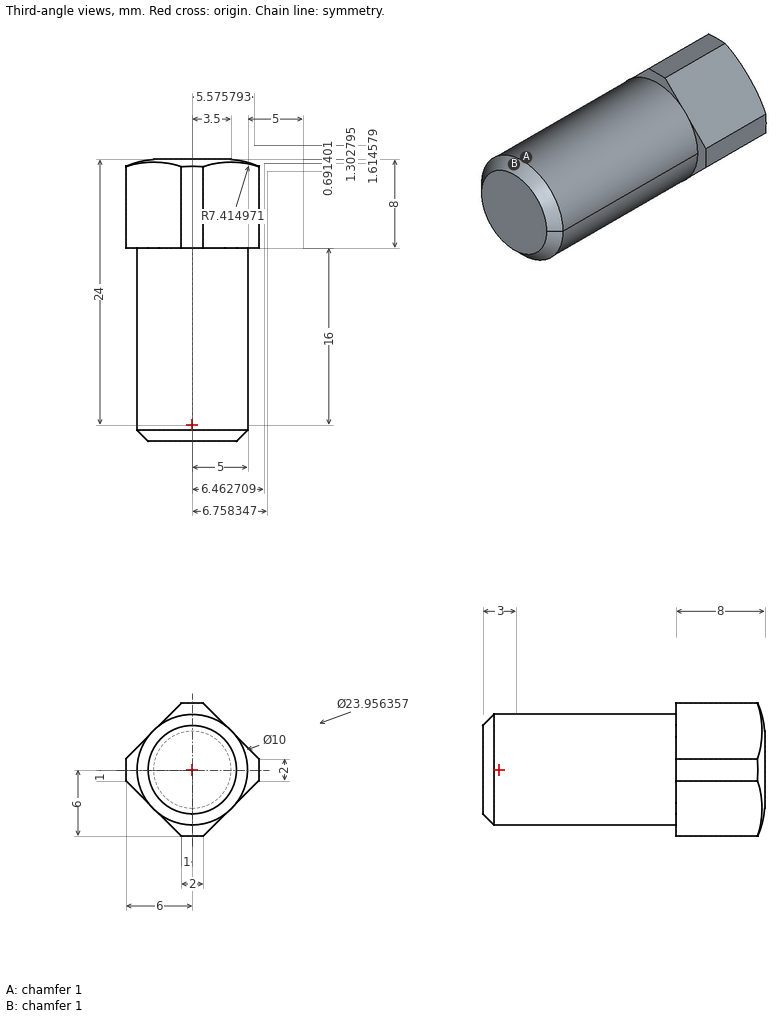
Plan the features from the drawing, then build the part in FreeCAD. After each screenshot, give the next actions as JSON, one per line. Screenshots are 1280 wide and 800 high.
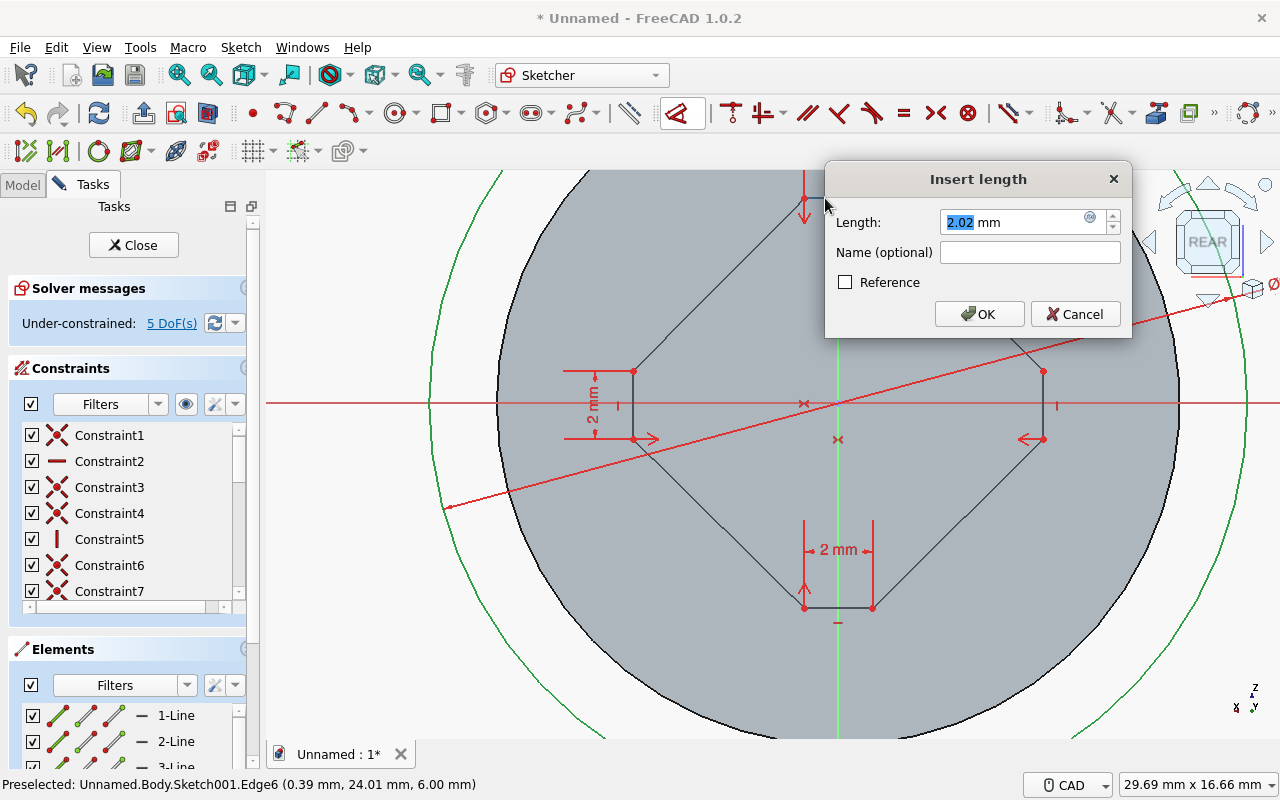
{"action": "type", "text": "2"}
{"action": "key", "text": "Return"}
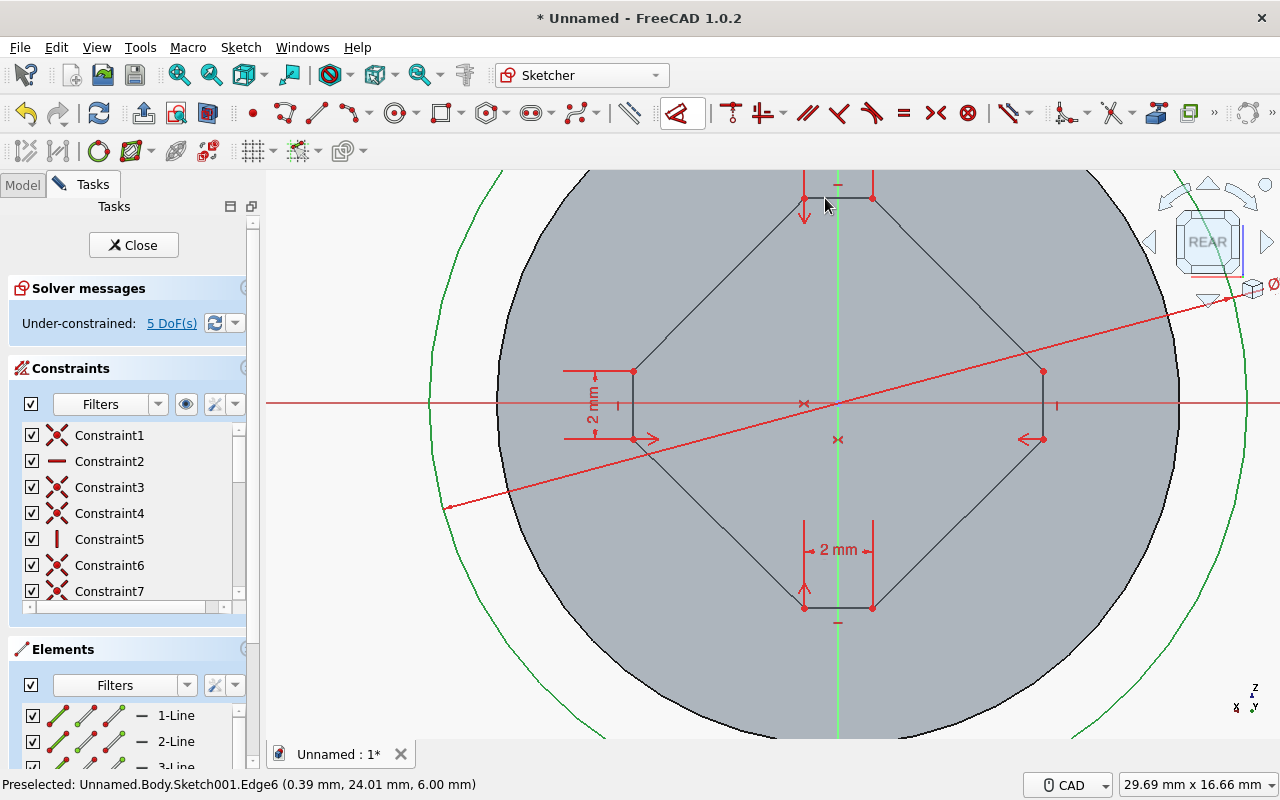
{"action": "left_click", "coordinate": [1043, 392]}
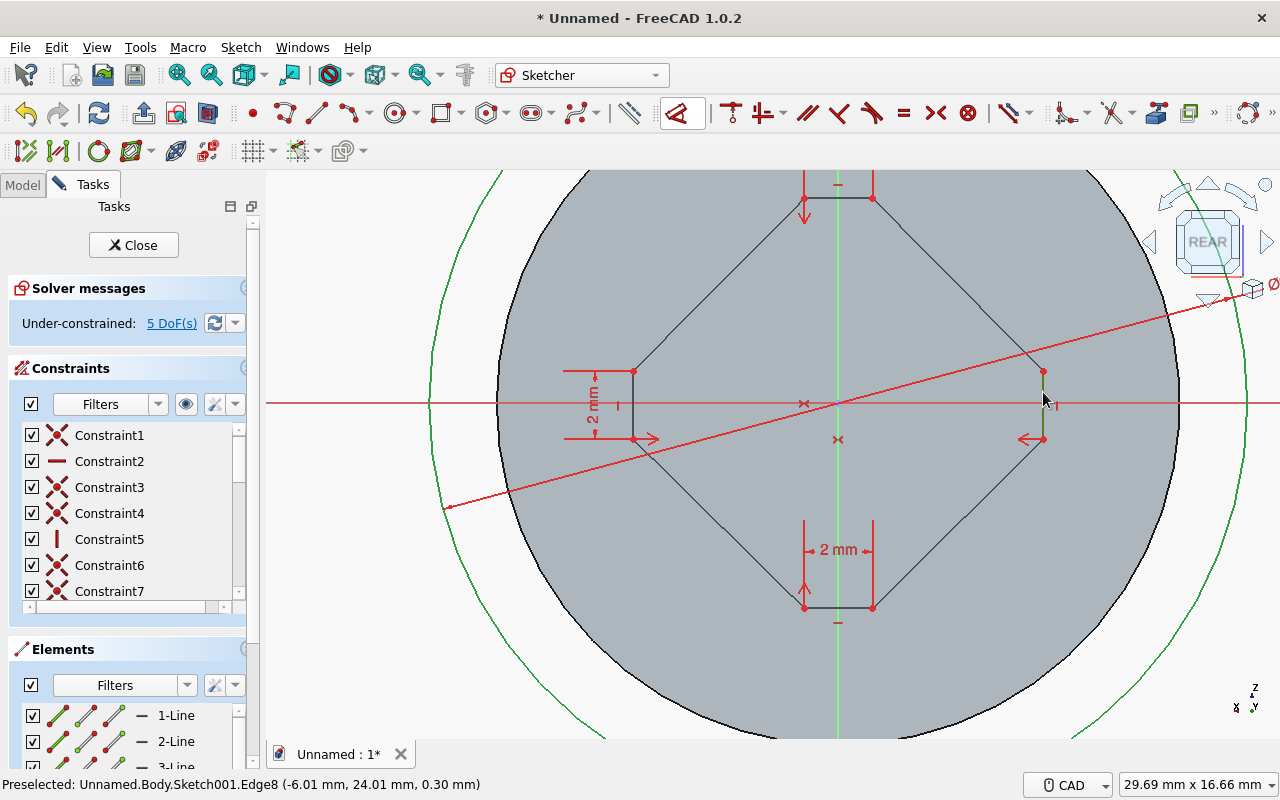
{"action": "key", "text": "i"}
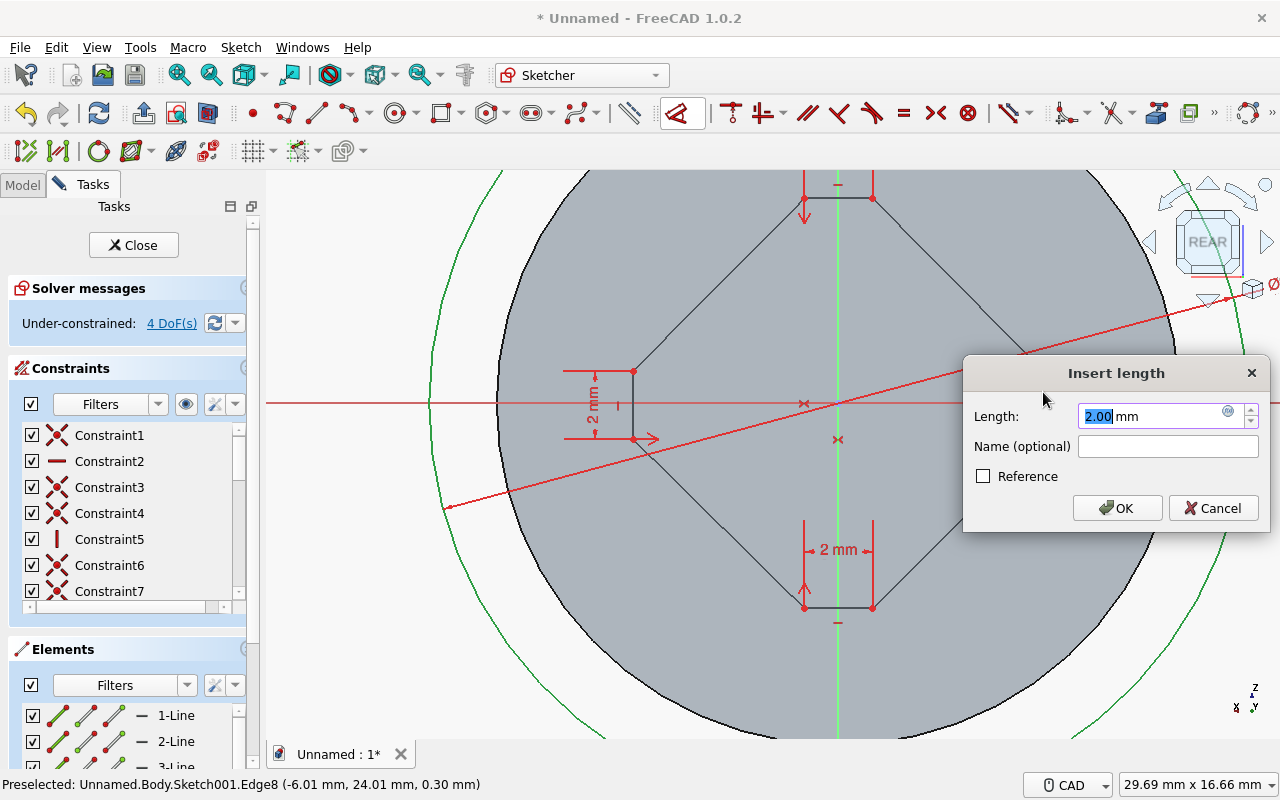
{"action": "type", "text": "2"}
{"action": "key", "text": "Return"}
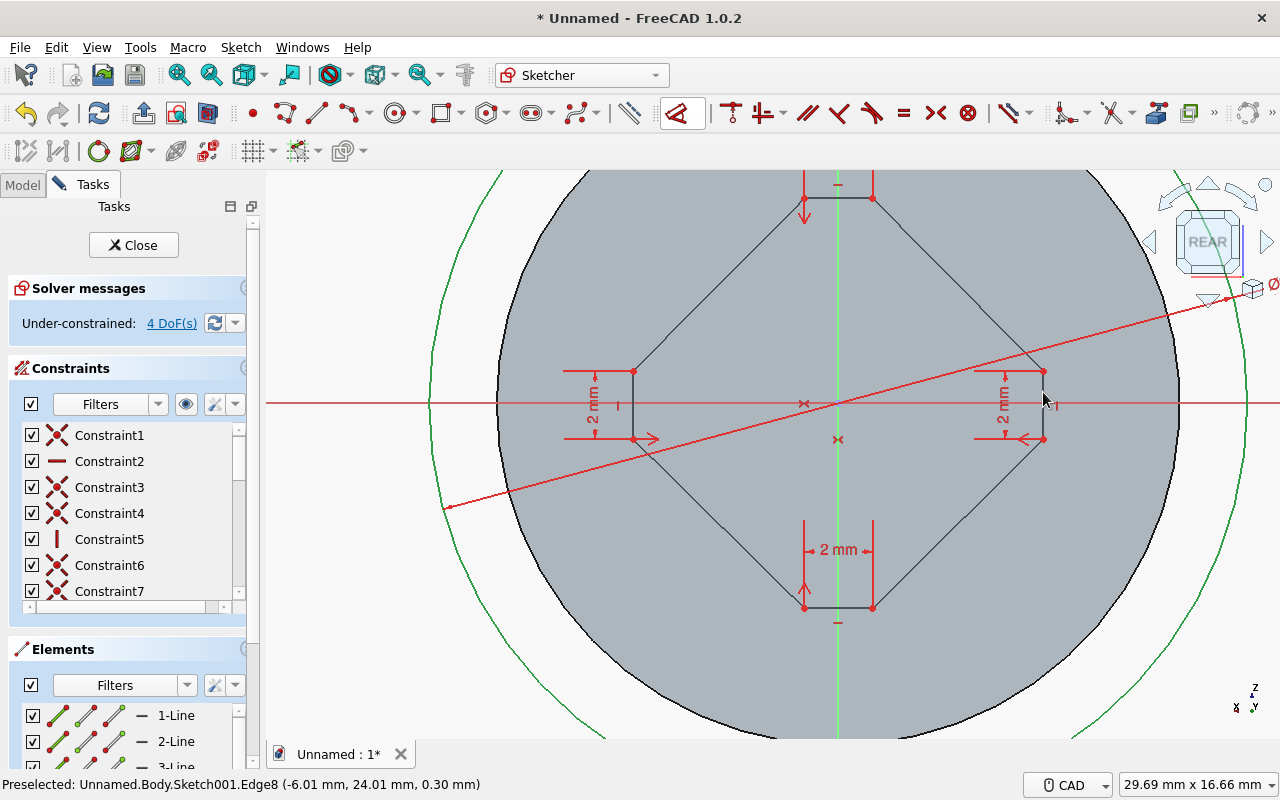
{"action": "left_click", "coordinate": [1043, 439]}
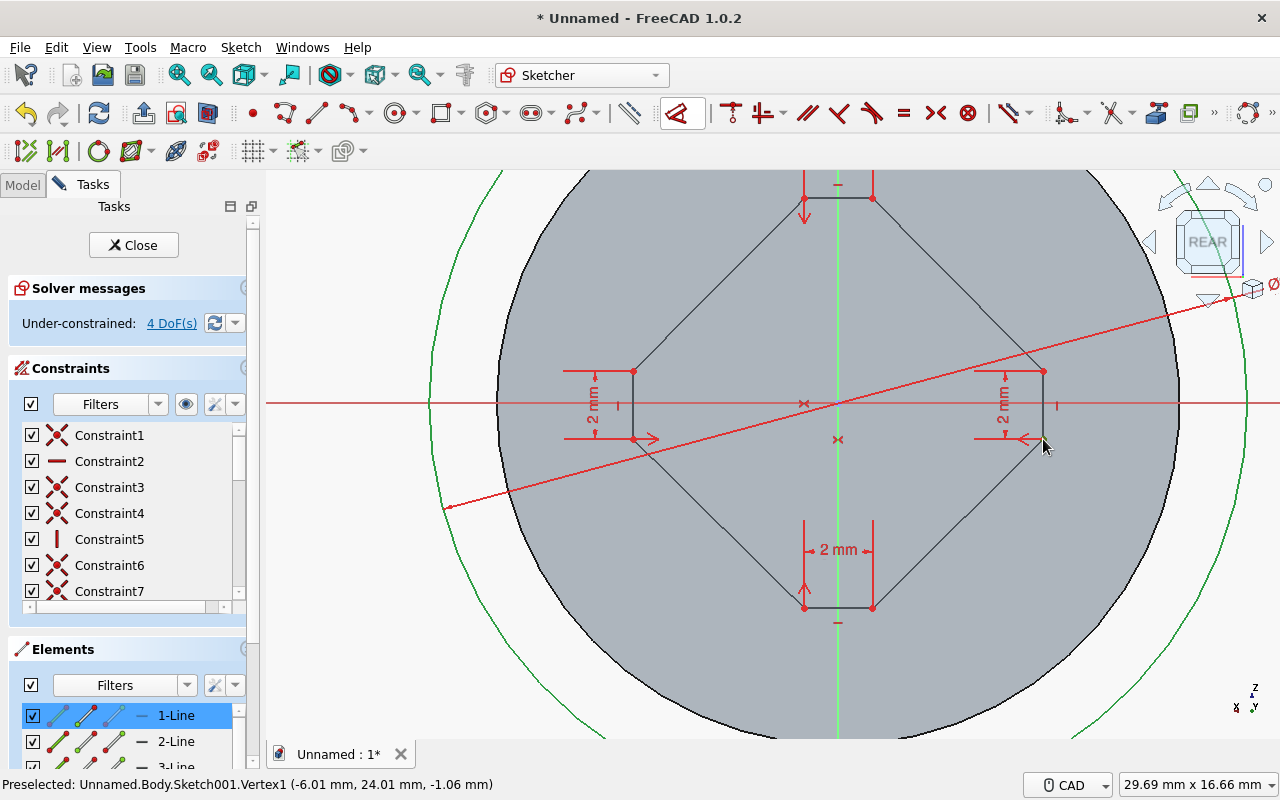
{"action": "left_click", "coordinate": [700, 114]}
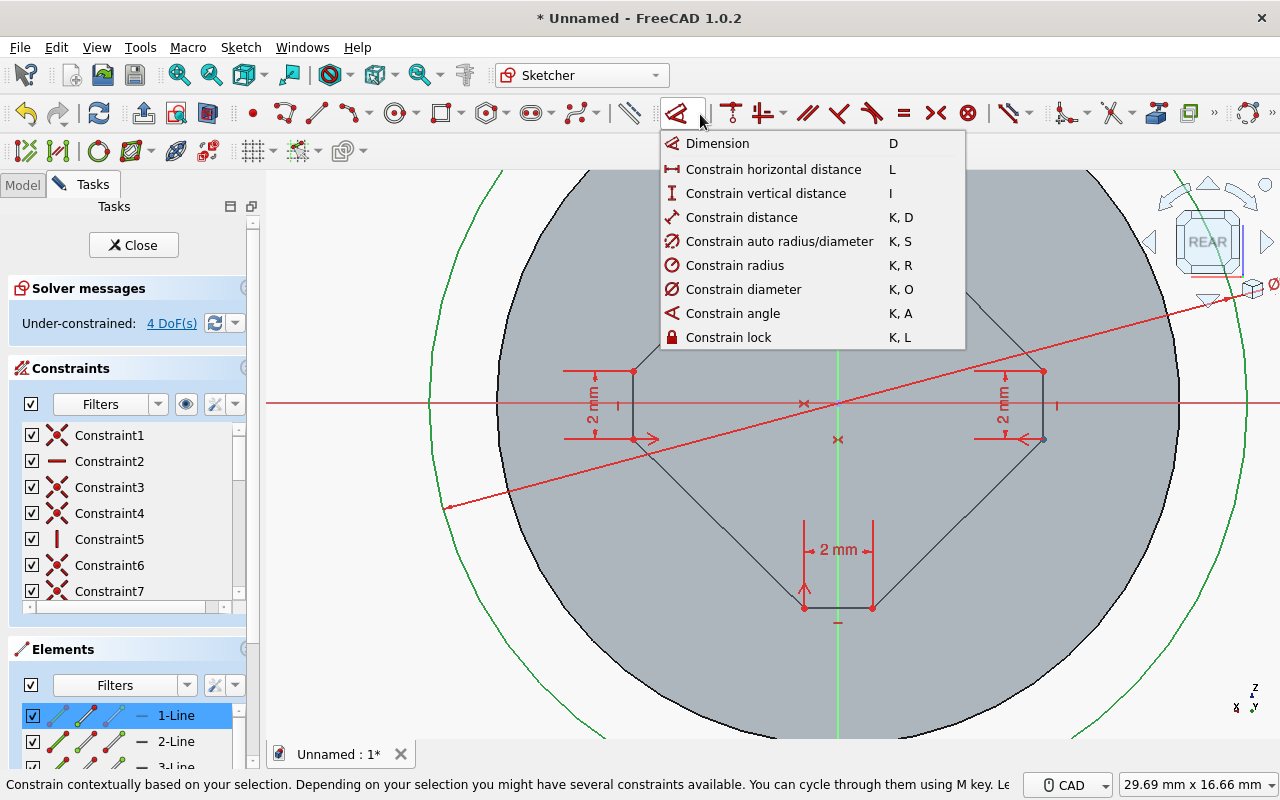
{"action": "left_click", "coordinate": [813, 169]}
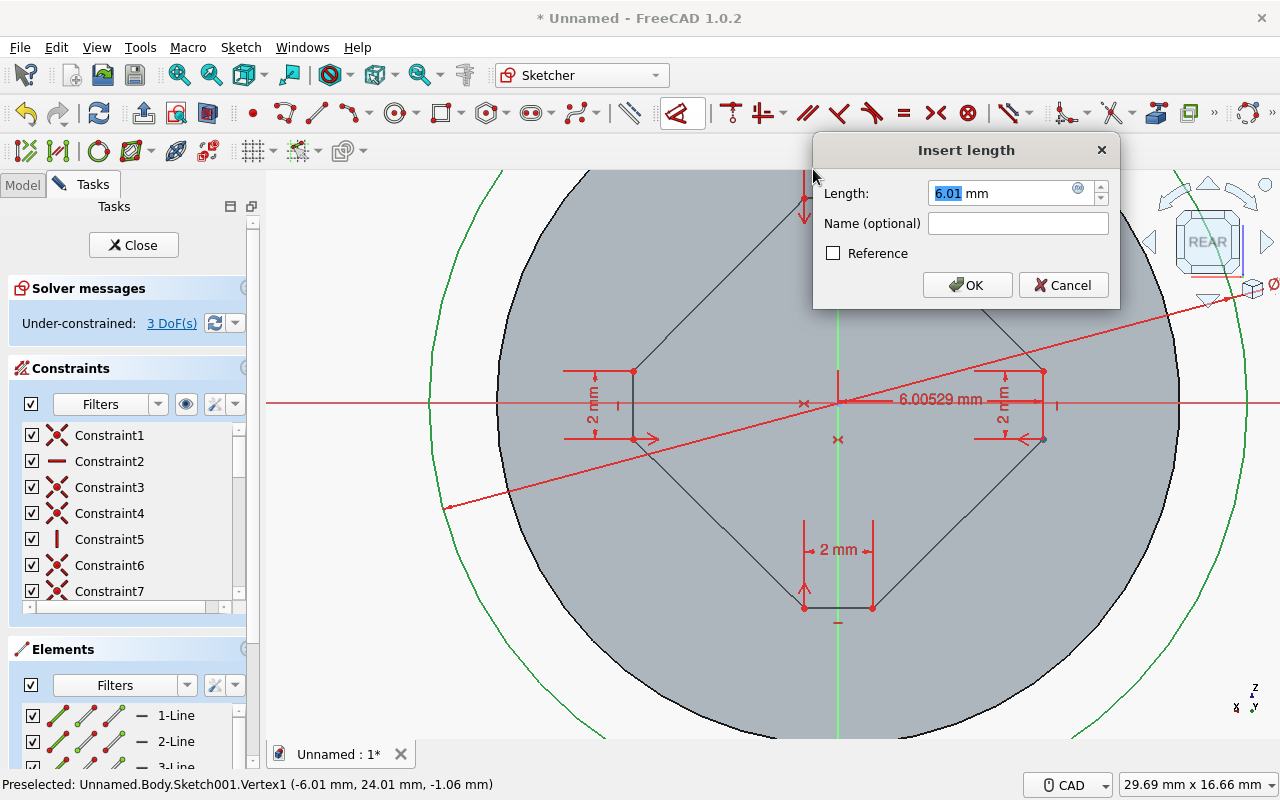
{"action": "type", "text": "6"}
{"action": "key", "text": "Return"}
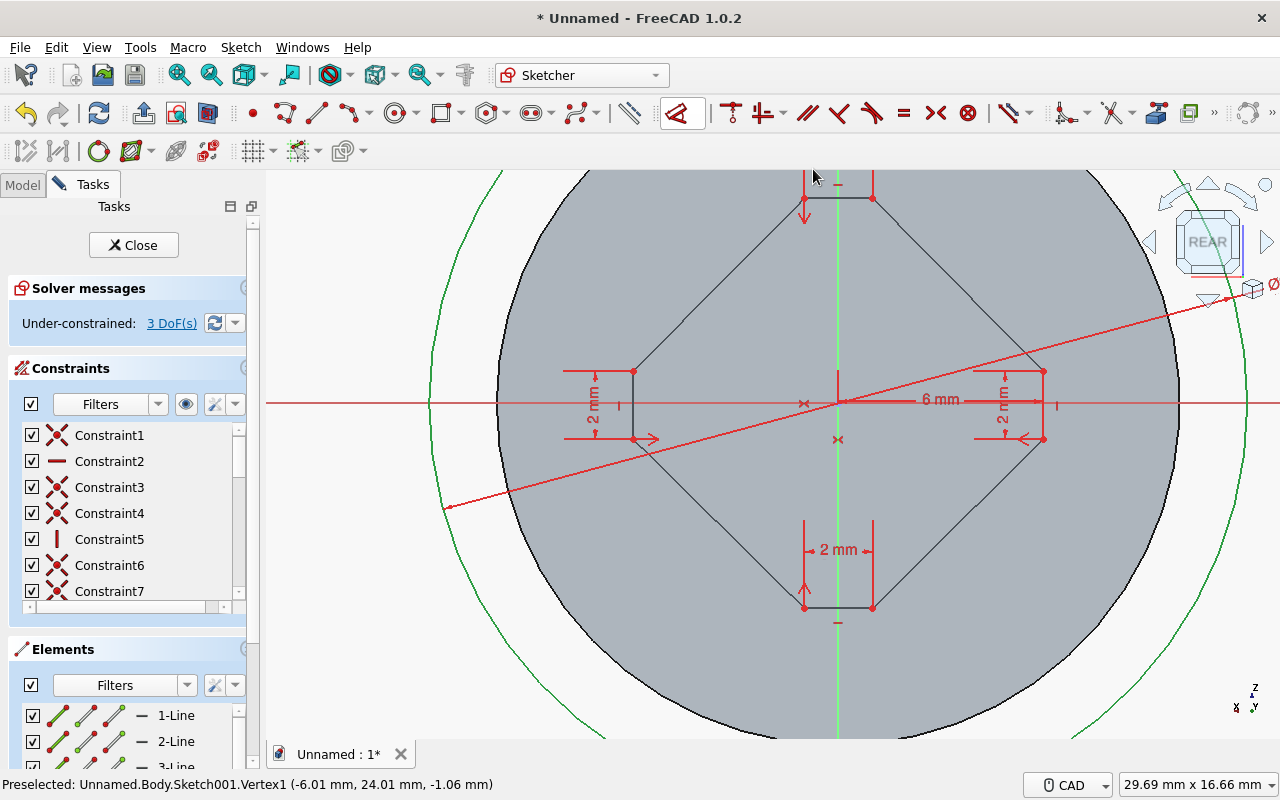
{"action": "left_click", "coordinate": [1043, 439]}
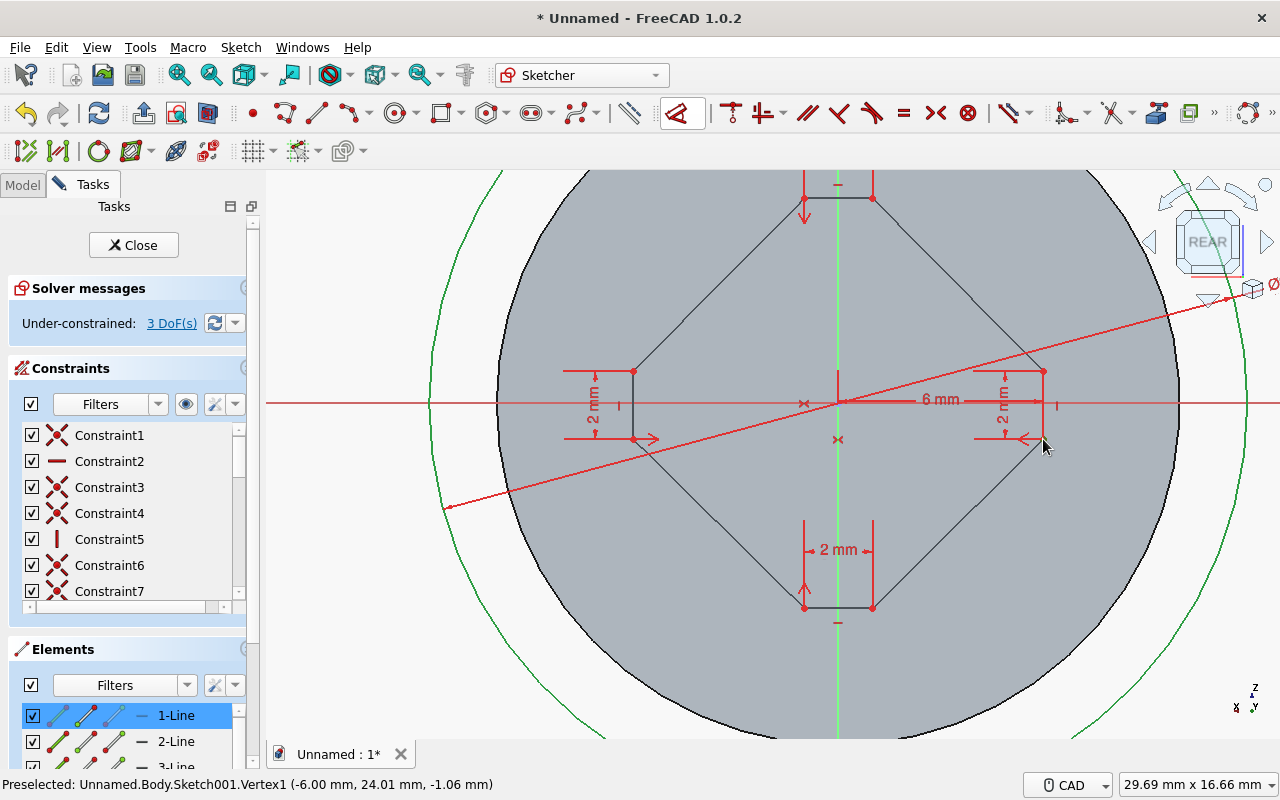
{"action": "key", "text": "i"}